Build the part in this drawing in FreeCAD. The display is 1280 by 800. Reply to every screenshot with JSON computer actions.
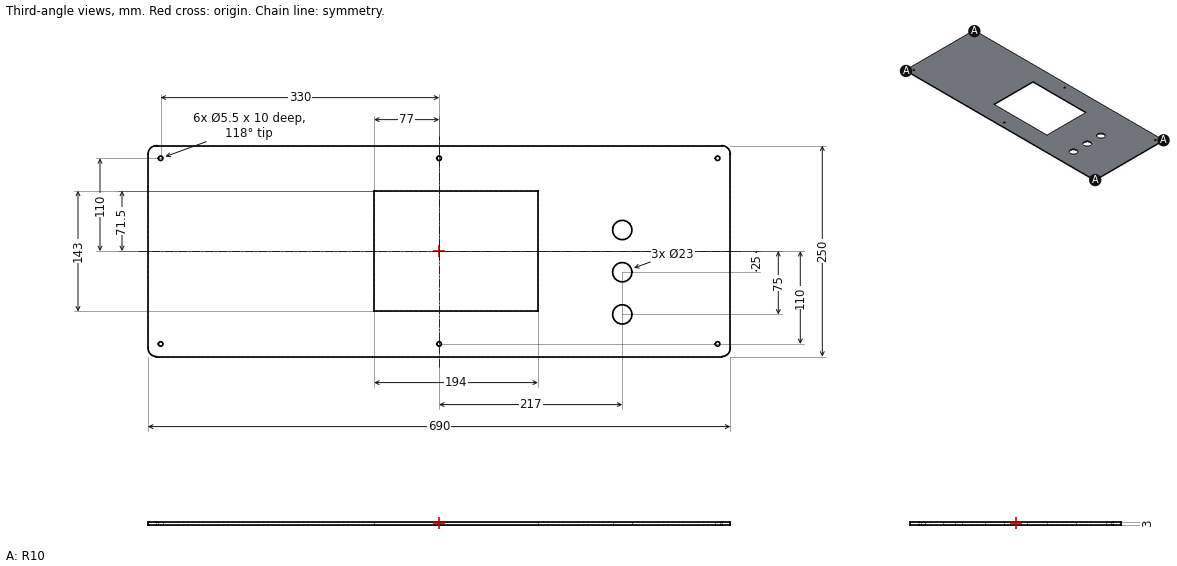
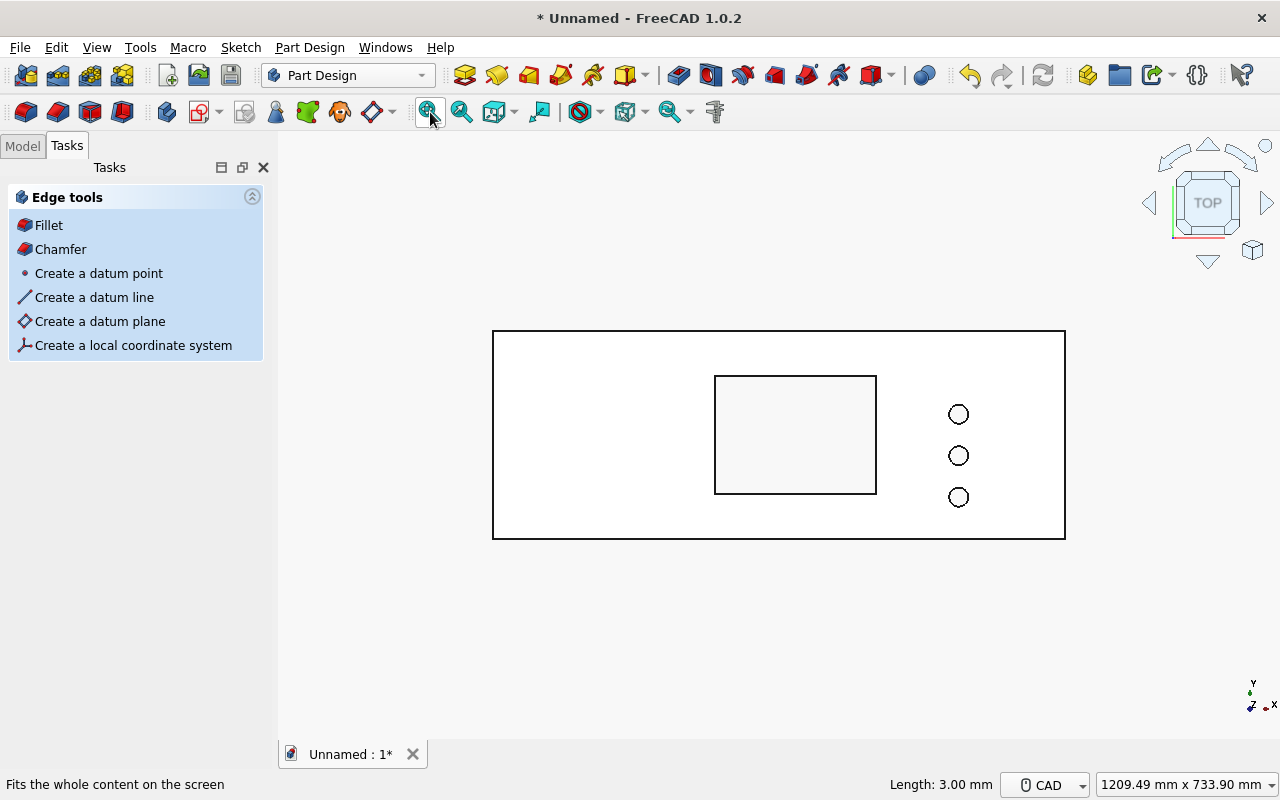
{"action": "key", "text": "1"}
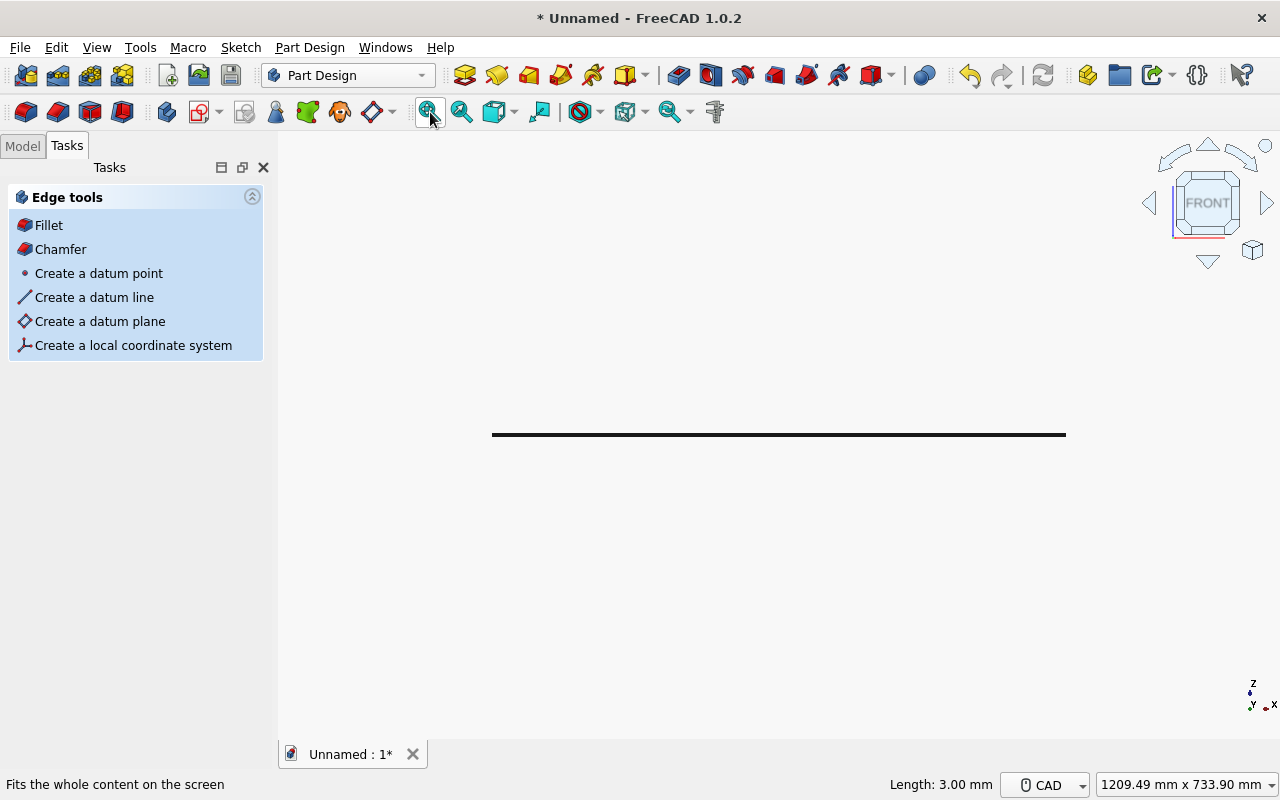
{"action": "scroll", "coordinate": [493, 434], "scroll_direction": "up", "scroll_amount": 14}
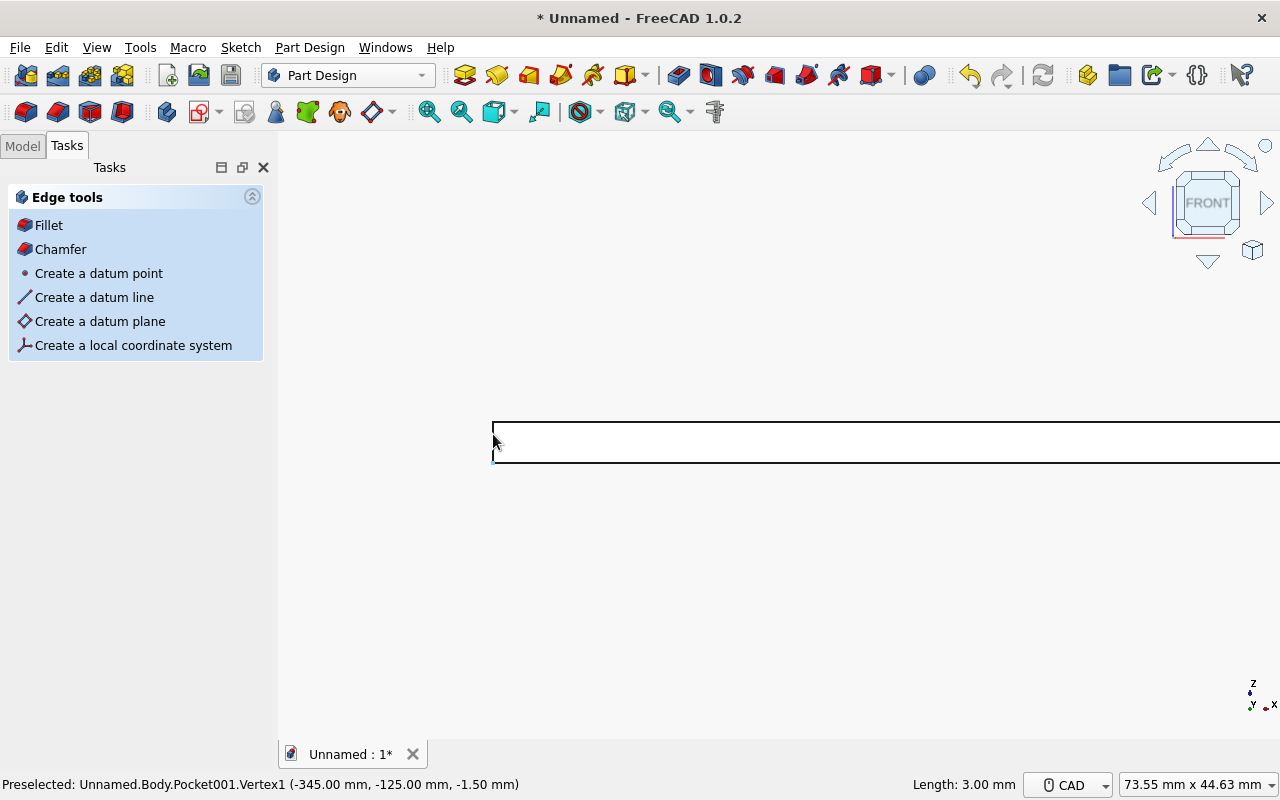
{"action": "left_click", "coordinate": [493, 442], "text": "ctrl"}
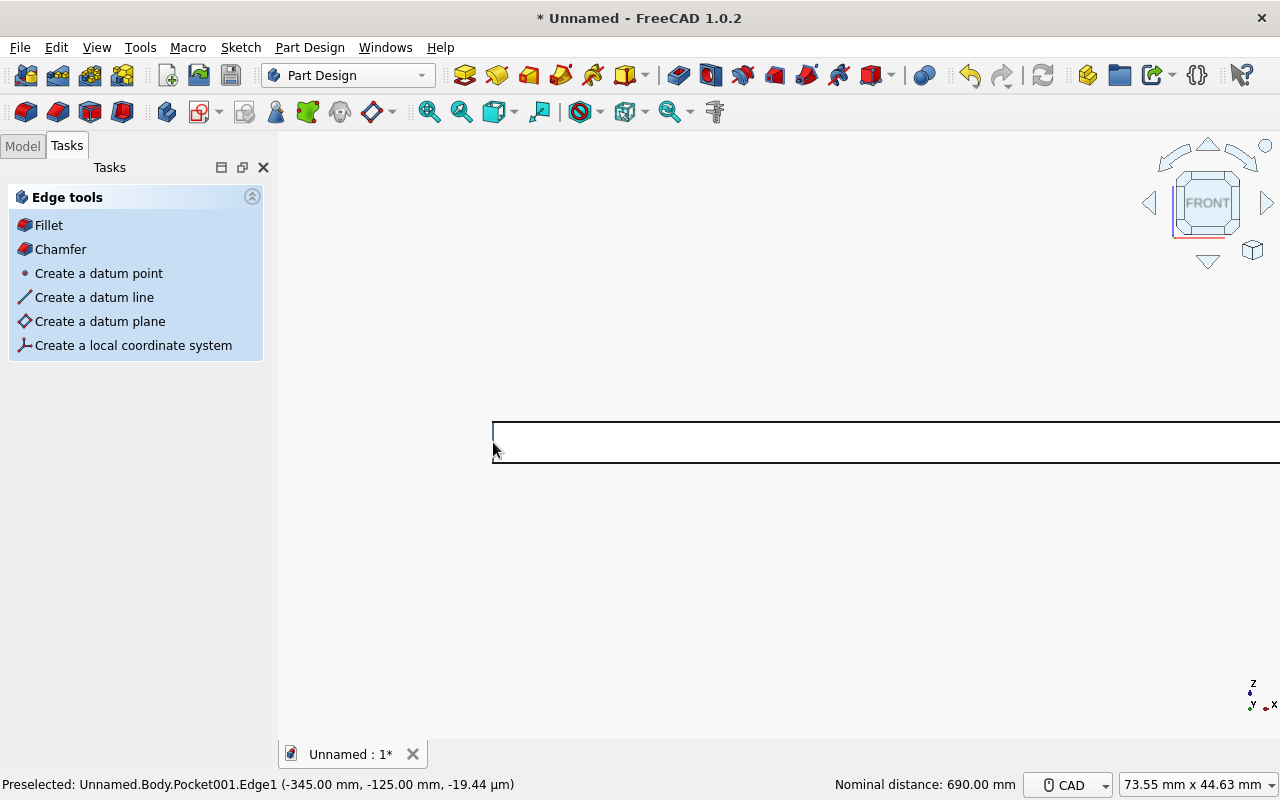
{"action": "left_click", "coordinate": [430, 112]}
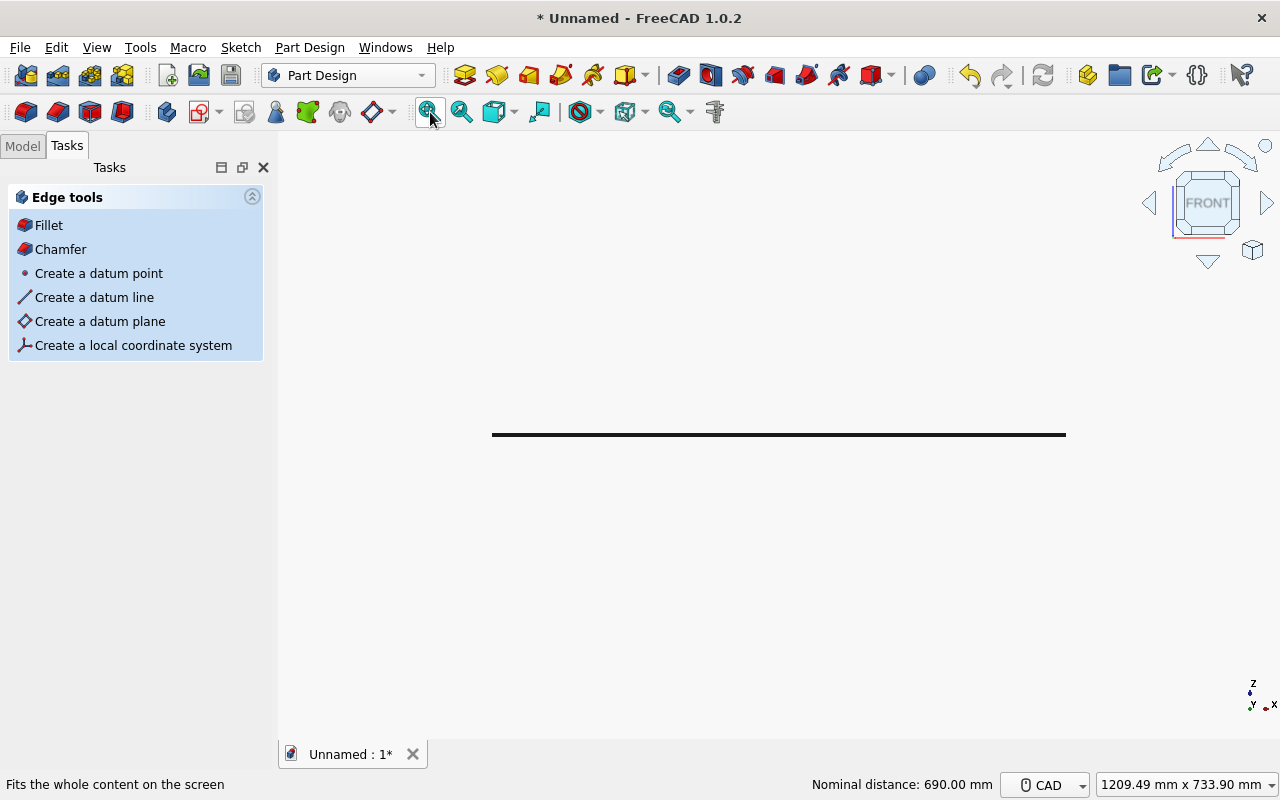
{"action": "key", "text": "3"}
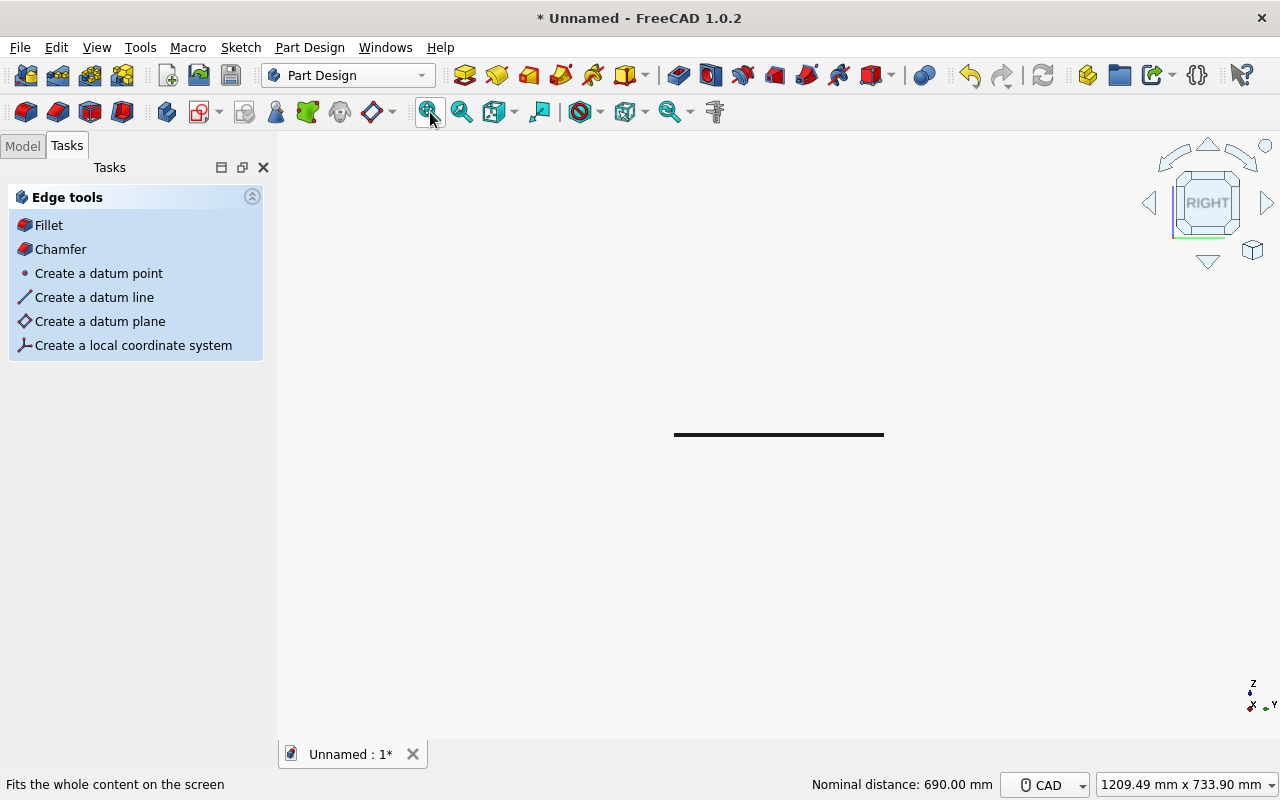
{"action": "left_click", "coordinate": [430, 112]}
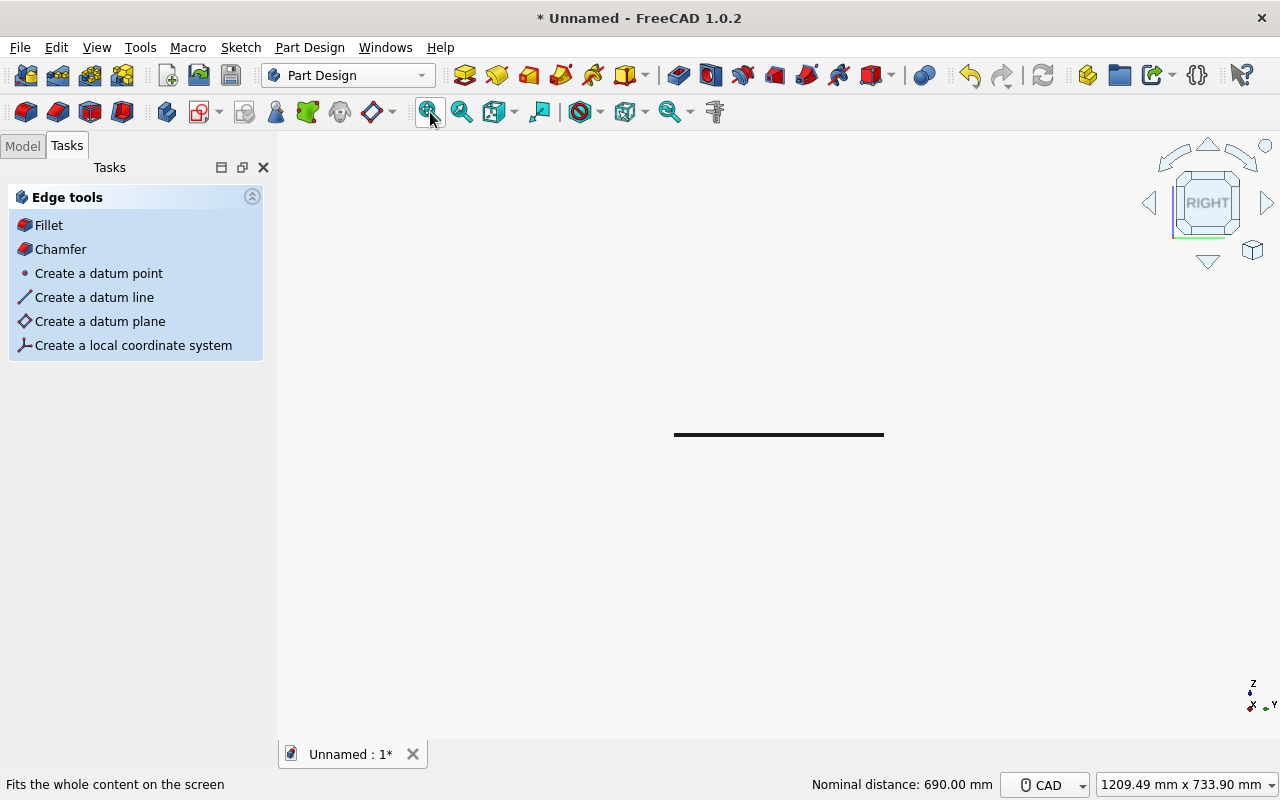
{"action": "scroll", "coordinate": [883, 434], "scroll_direction": "up", "scroll_amount": 14}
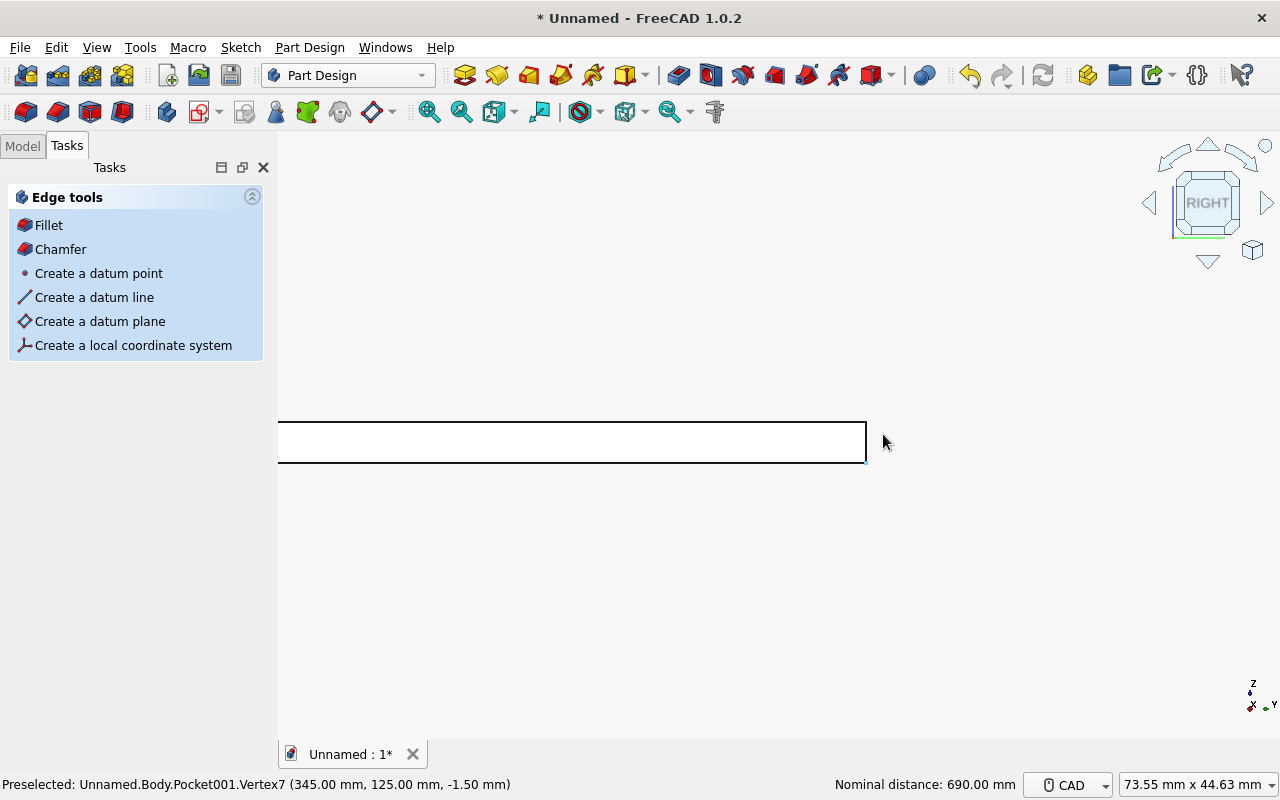
{"action": "left_click", "coordinate": [866, 442], "text": "ctrl"}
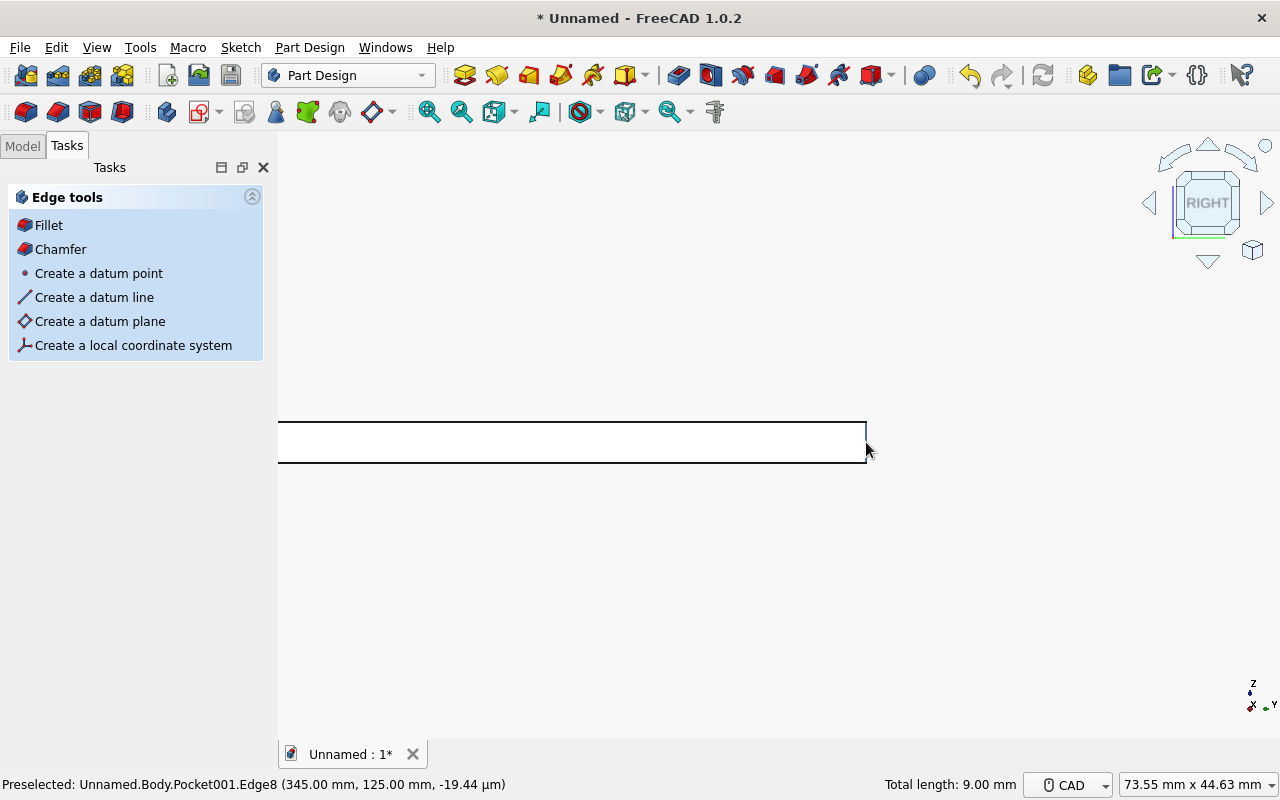
{"action": "left_click", "coordinate": [430, 112]}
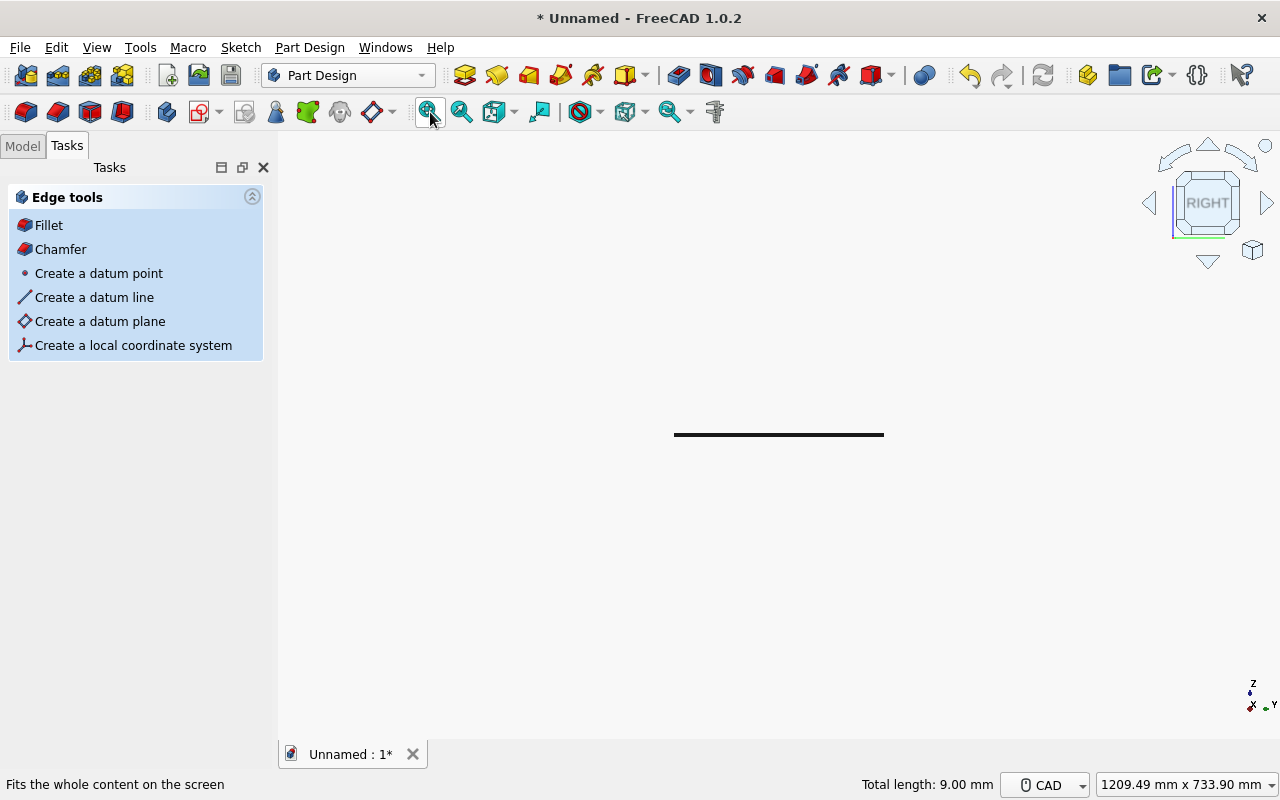
{"action": "key", "text": "5"}